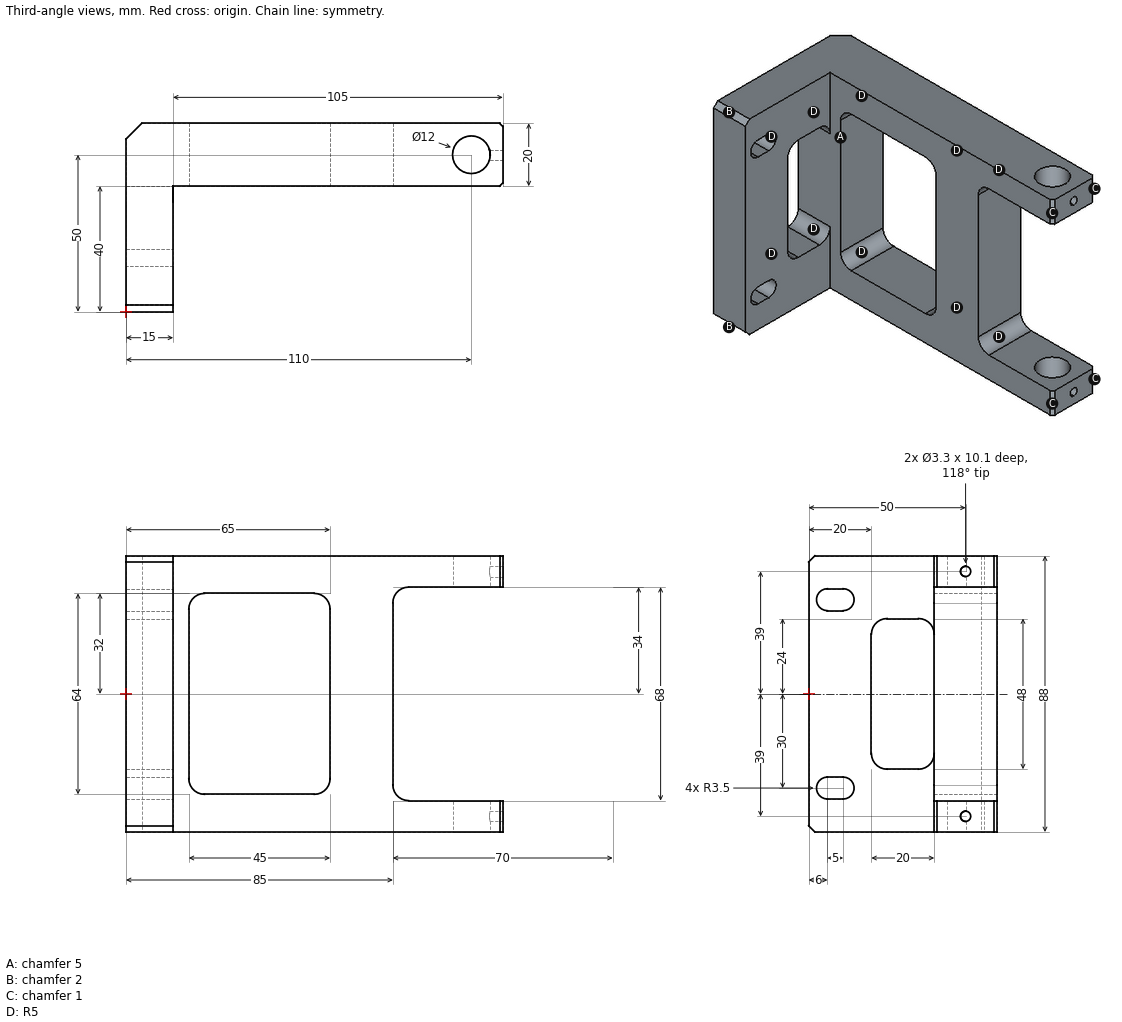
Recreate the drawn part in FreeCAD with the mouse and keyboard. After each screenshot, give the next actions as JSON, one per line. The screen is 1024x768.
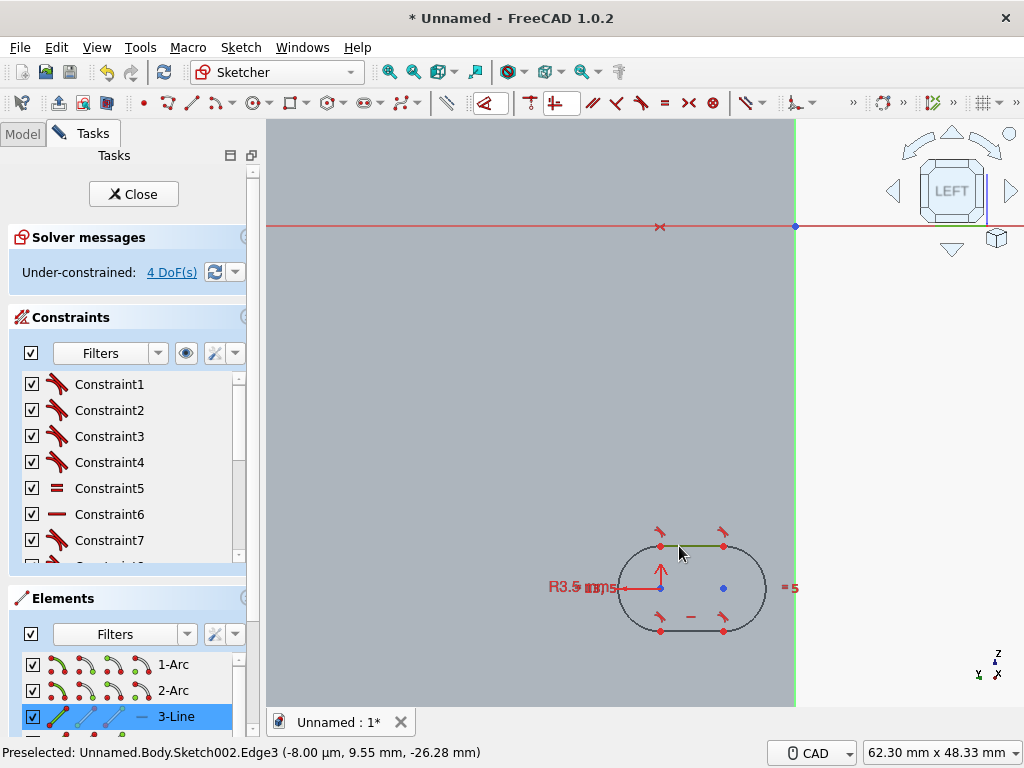
{"action": "key", "text": "l"}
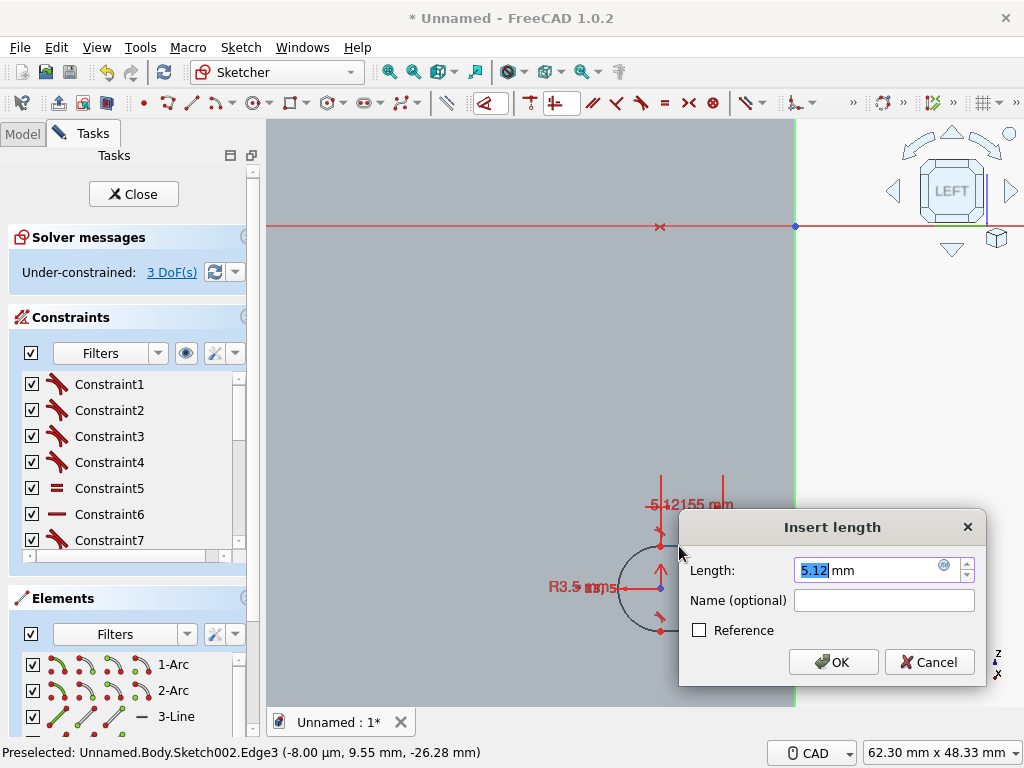
{"action": "type", "text": "5"}
{"action": "key", "text": "Return"}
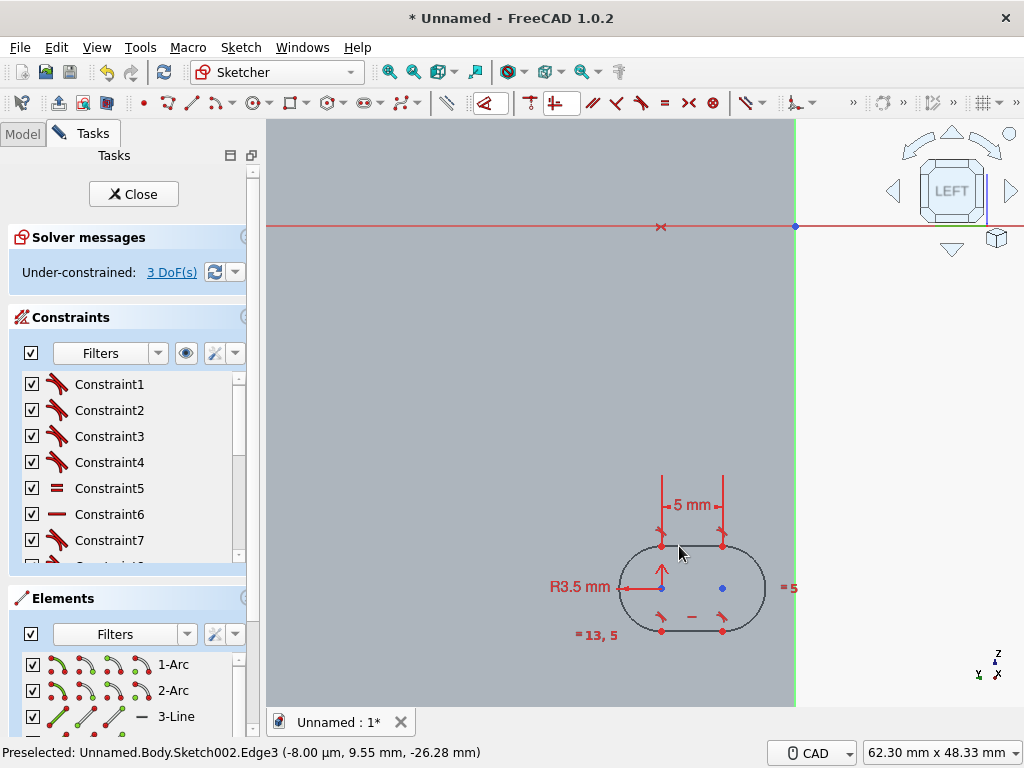
{"action": "scroll", "coordinate": [470, 565], "scroll_direction": "down", "scroll_amount": 4}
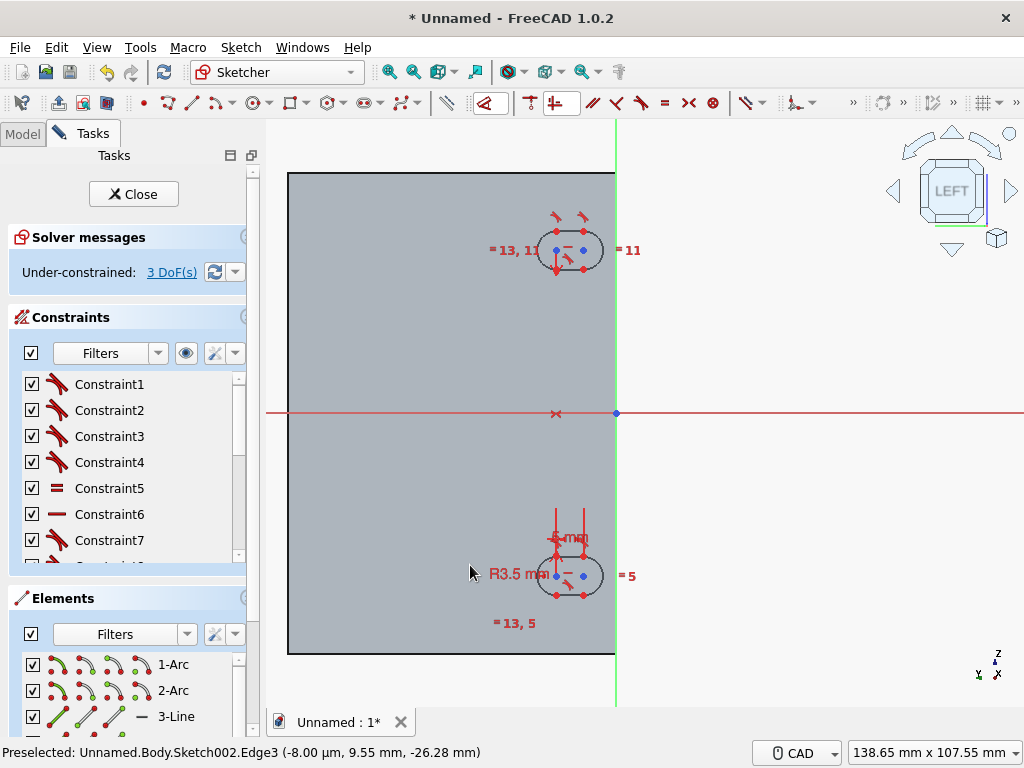
{"action": "scroll", "coordinate": [565, 231], "scroll_direction": "up", "scroll_amount": 3}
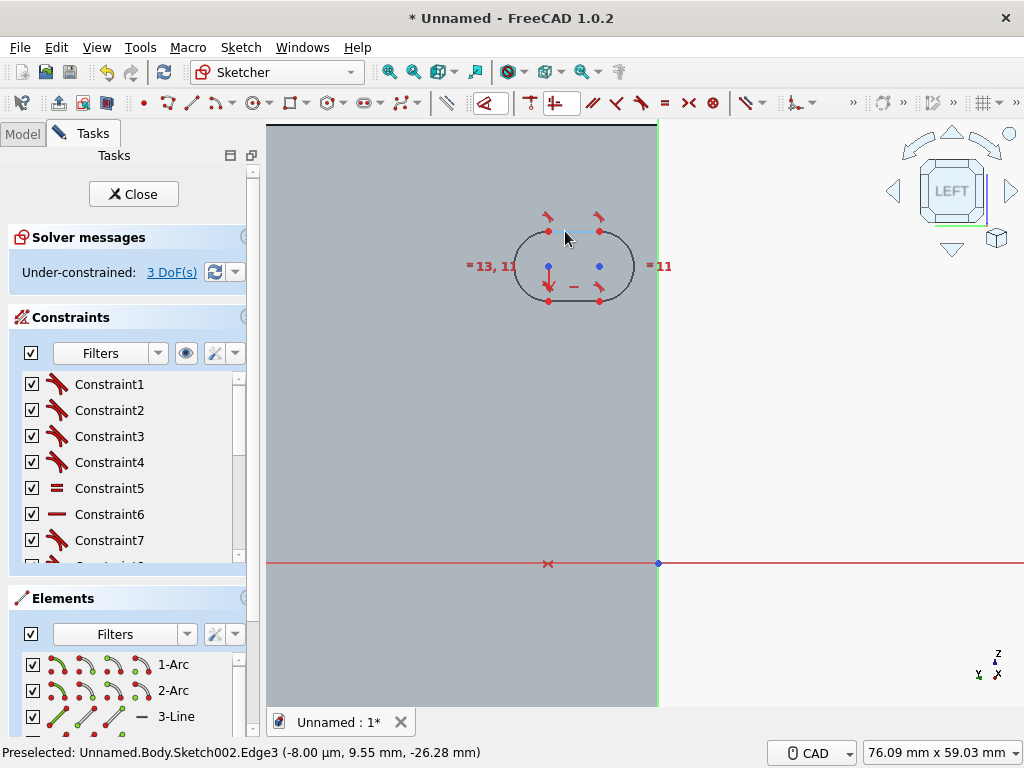
{"action": "left_click", "coordinate": [564, 232]}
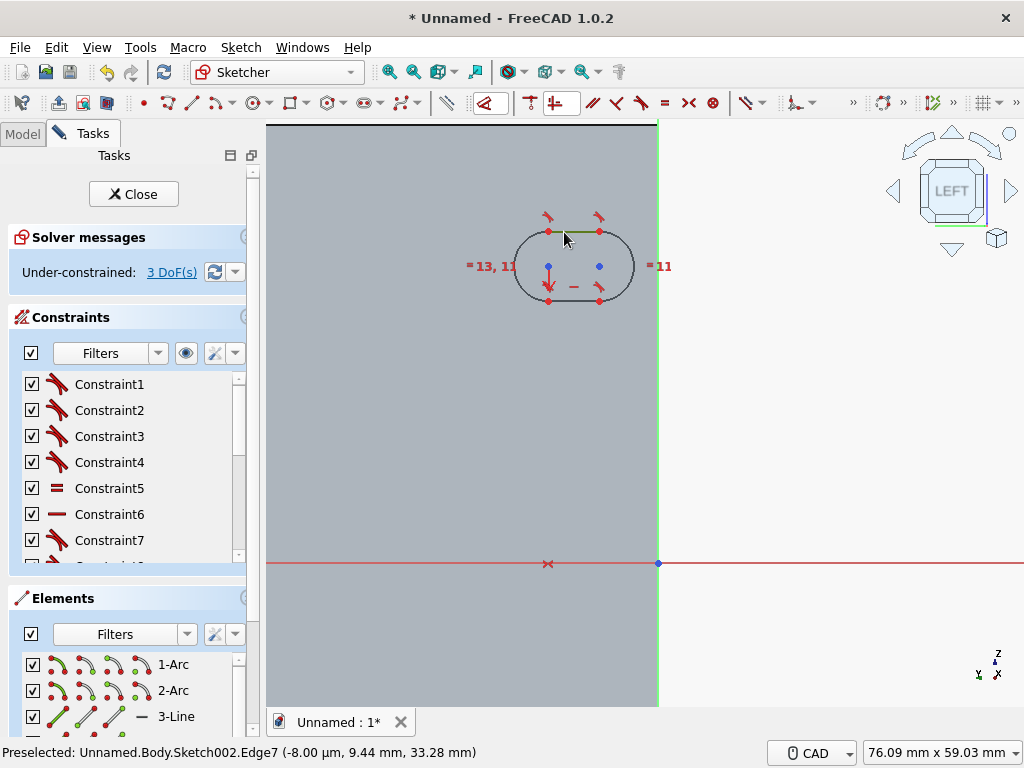
{"action": "key", "text": "l"}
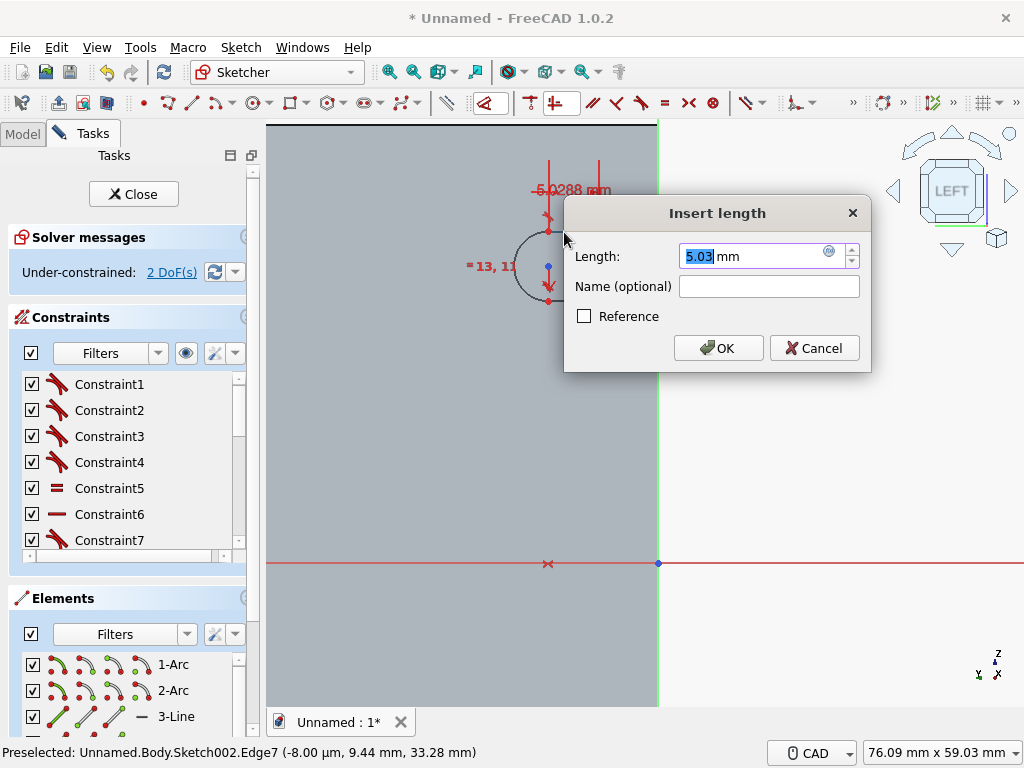
{"action": "type", "text": "5"}
{"action": "key", "text": "Return"}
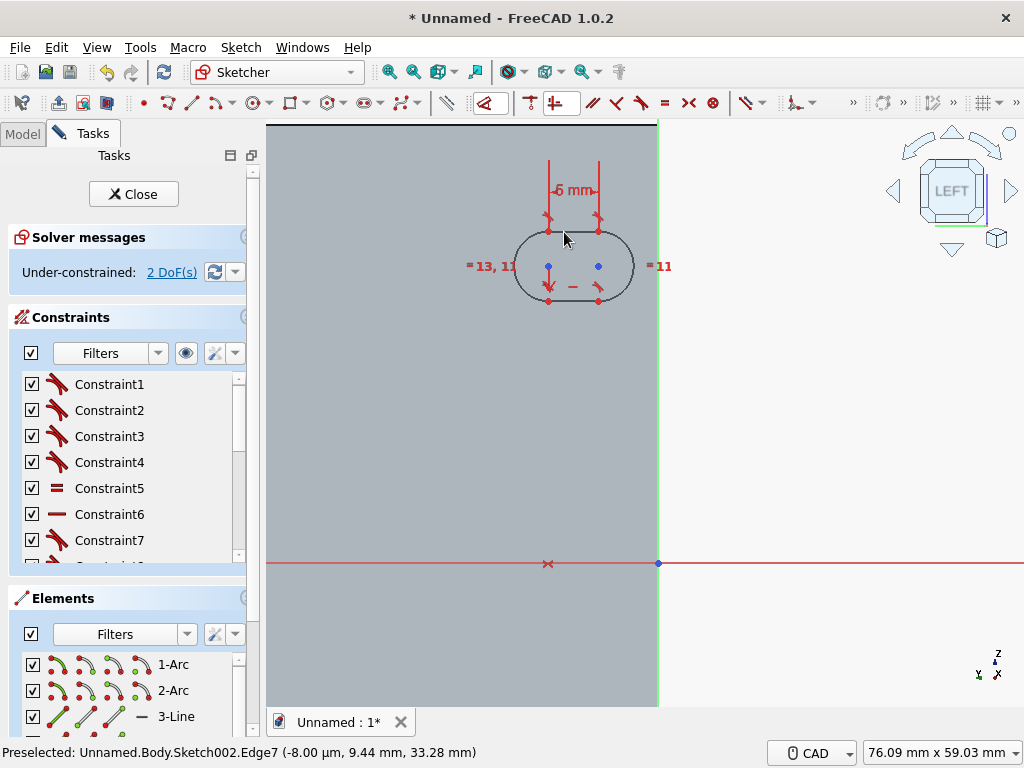
{"action": "scroll", "coordinate": [565, 231], "scroll_direction": "down", "scroll_amount": 3}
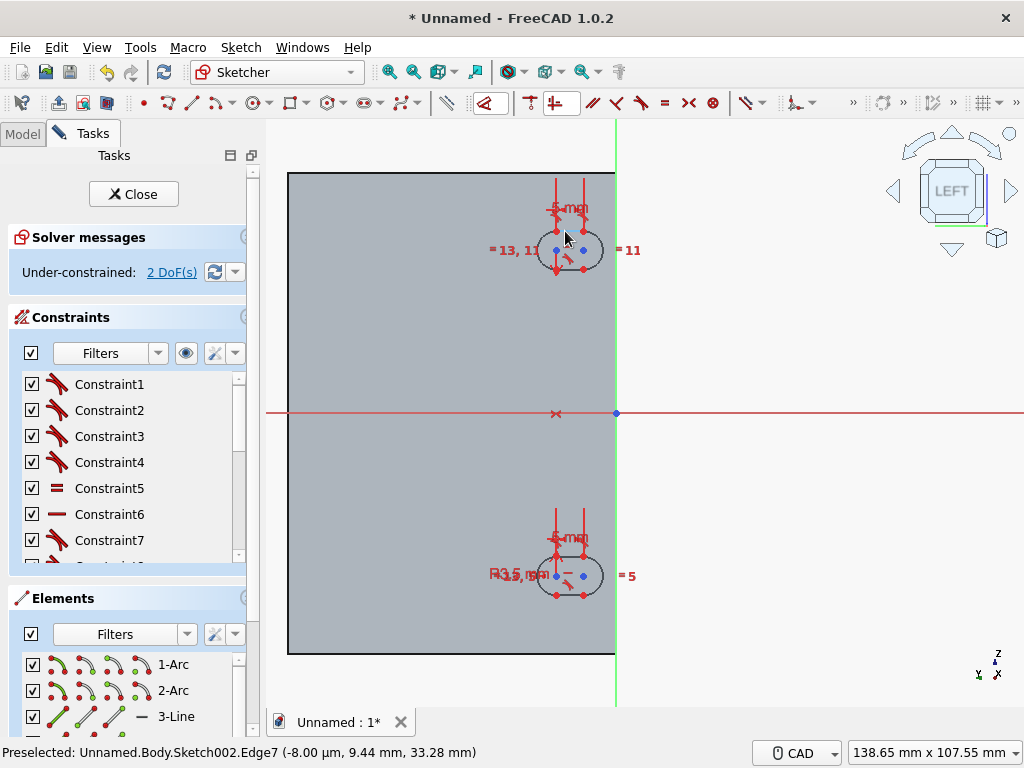
{"action": "left_click", "coordinate": [584, 595]}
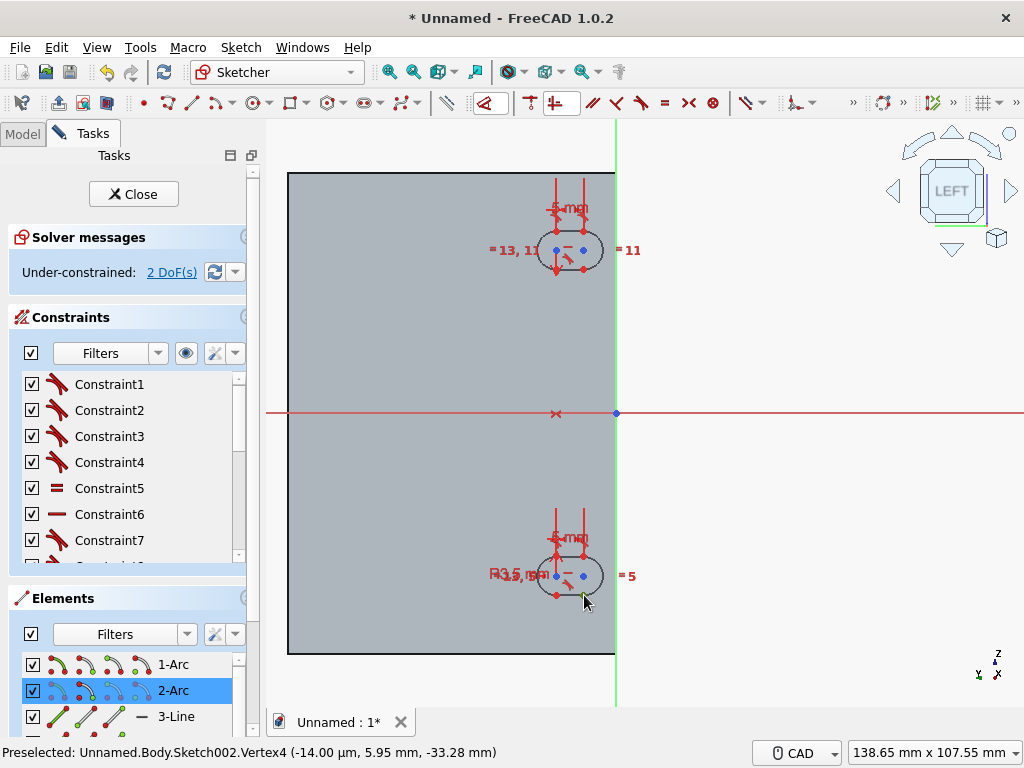
{"action": "key", "text": "l"}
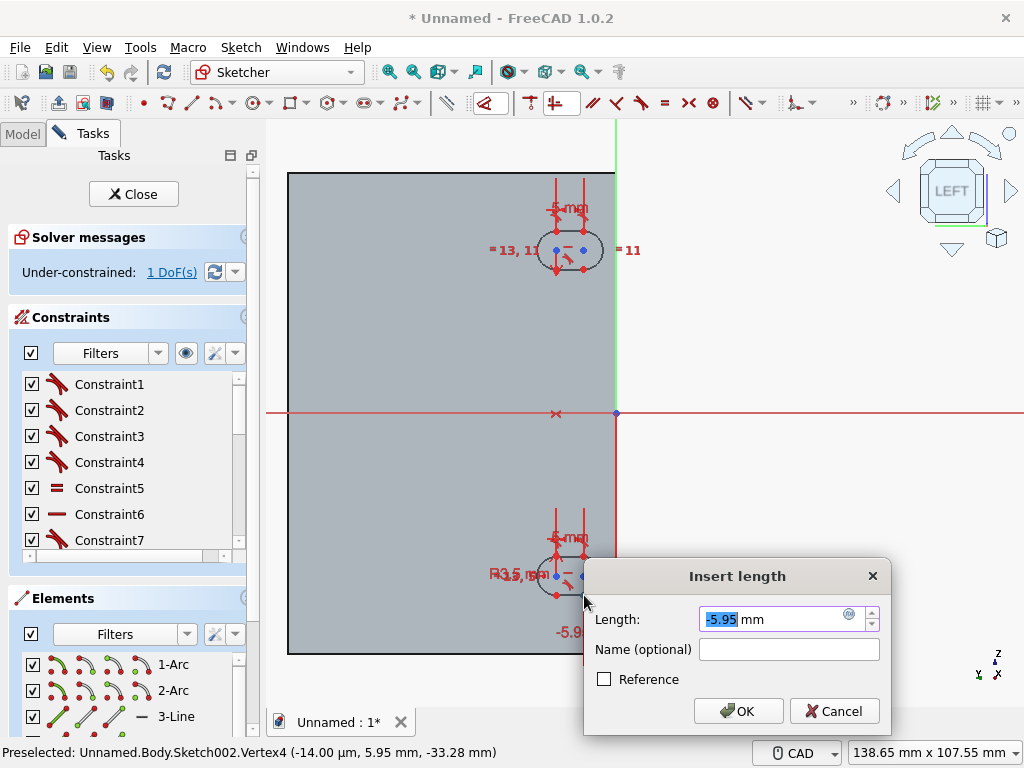
{"action": "type", "text": "-6"}
{"action": "key", "text": "Return"}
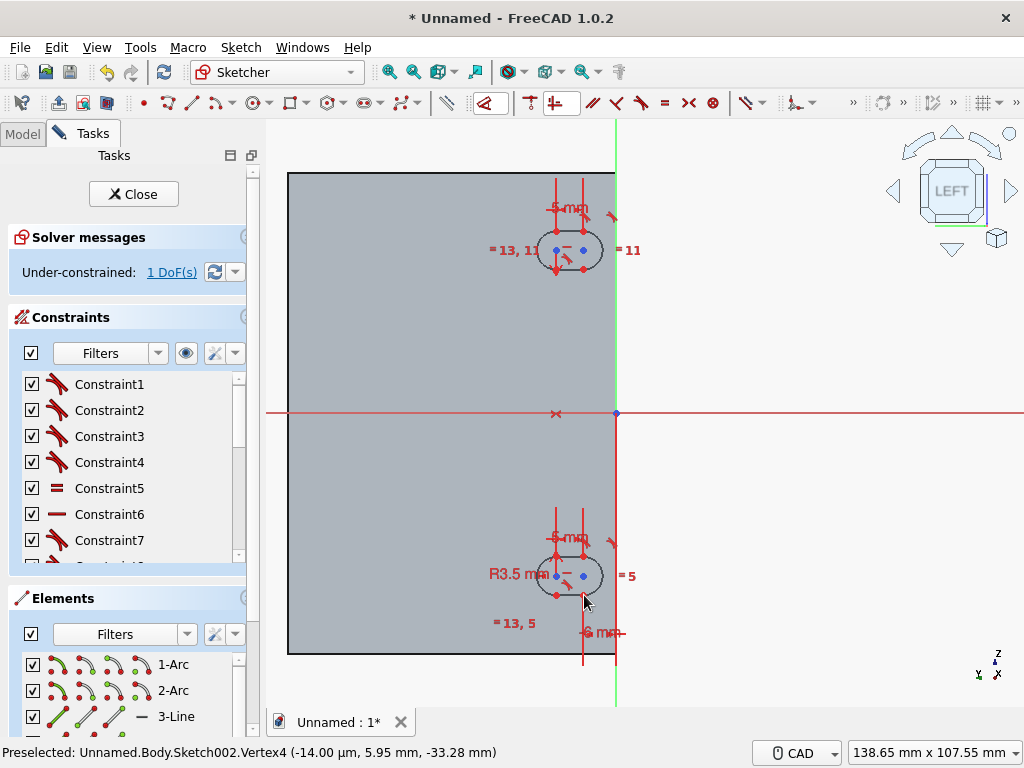
{"action": "left_click", "coordinate": [556, 576]}